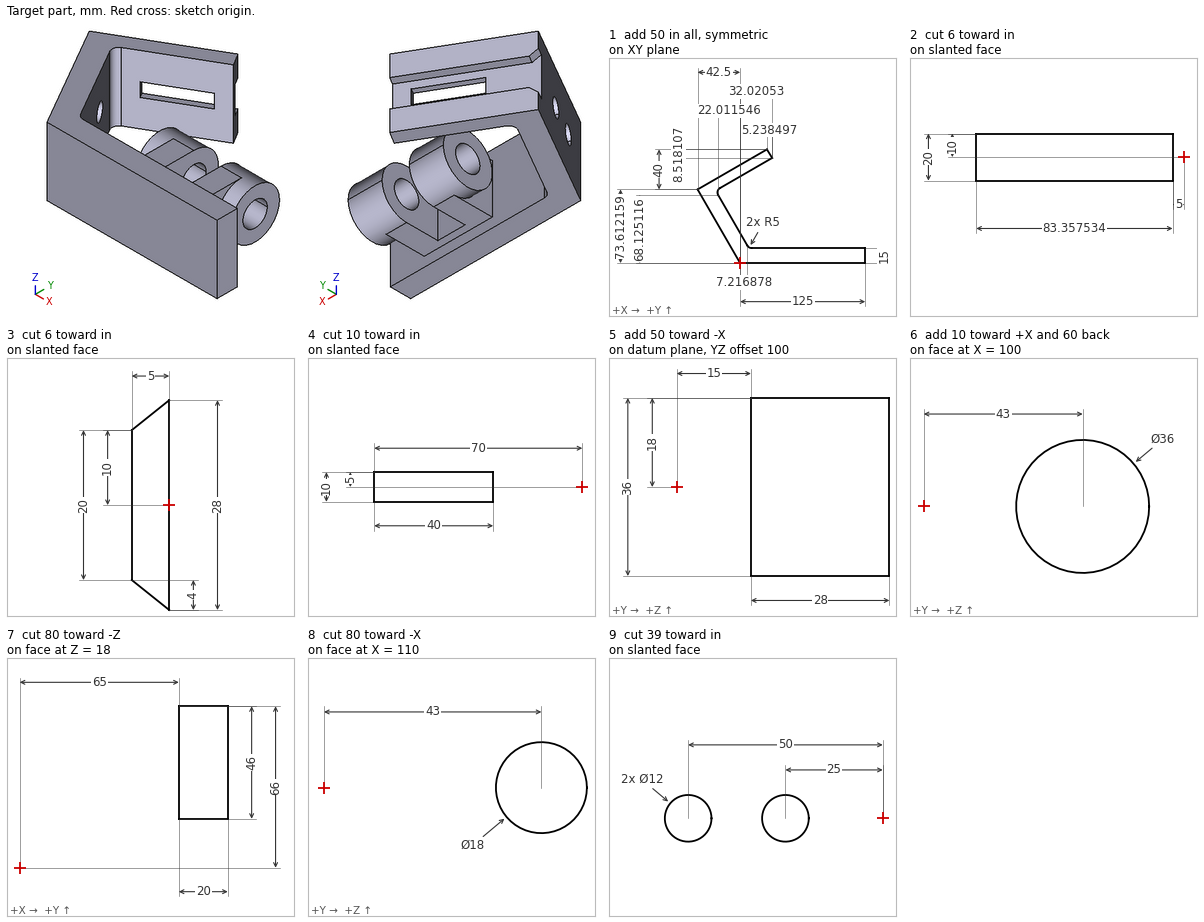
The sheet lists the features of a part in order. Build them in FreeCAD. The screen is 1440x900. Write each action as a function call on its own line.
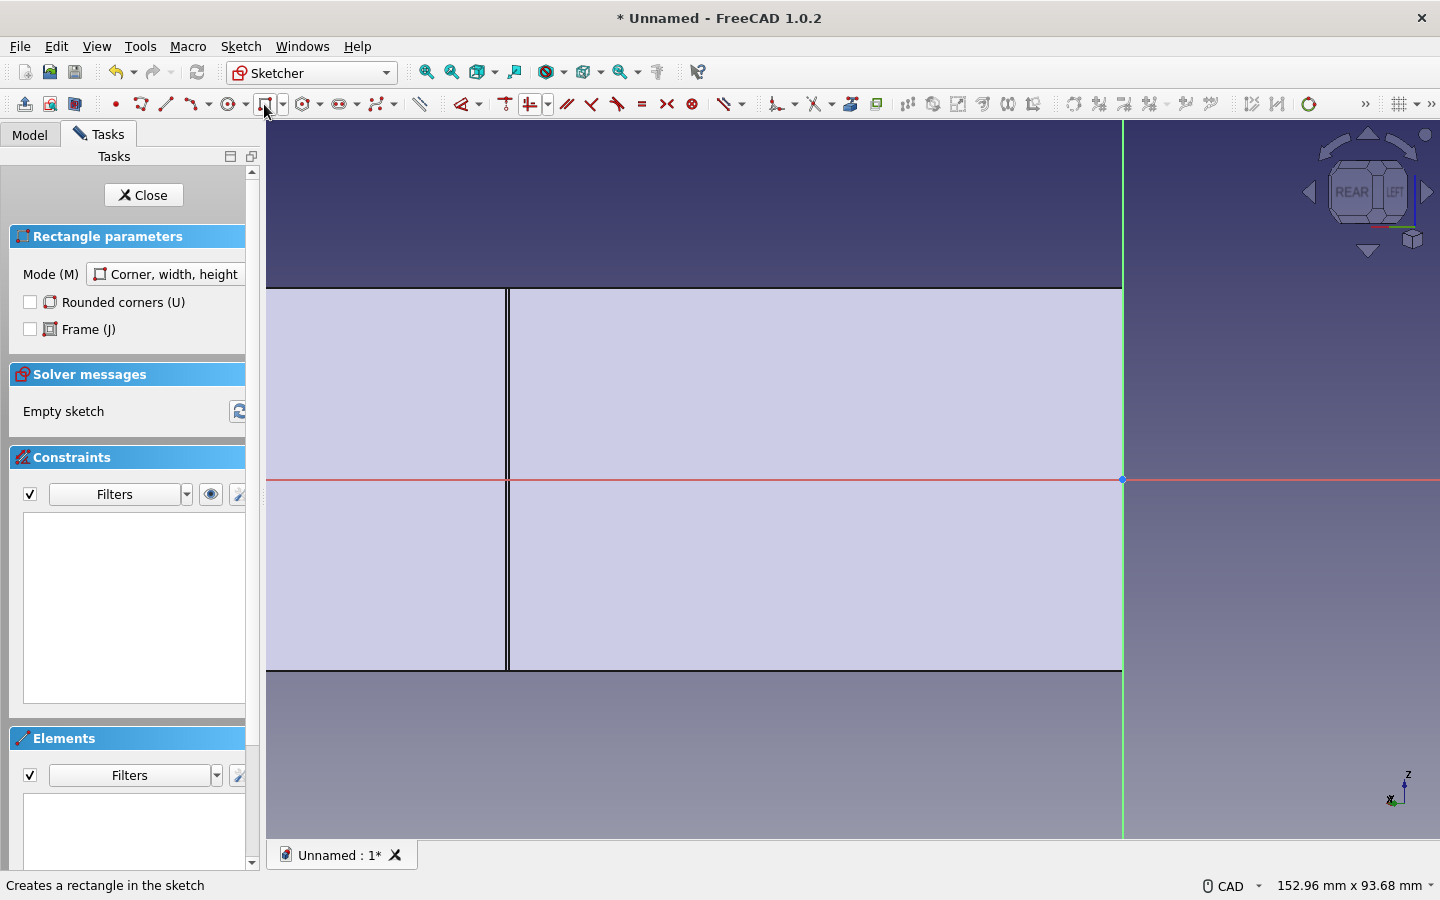
click(444, 403)
click(1084, 556)
key(Escape)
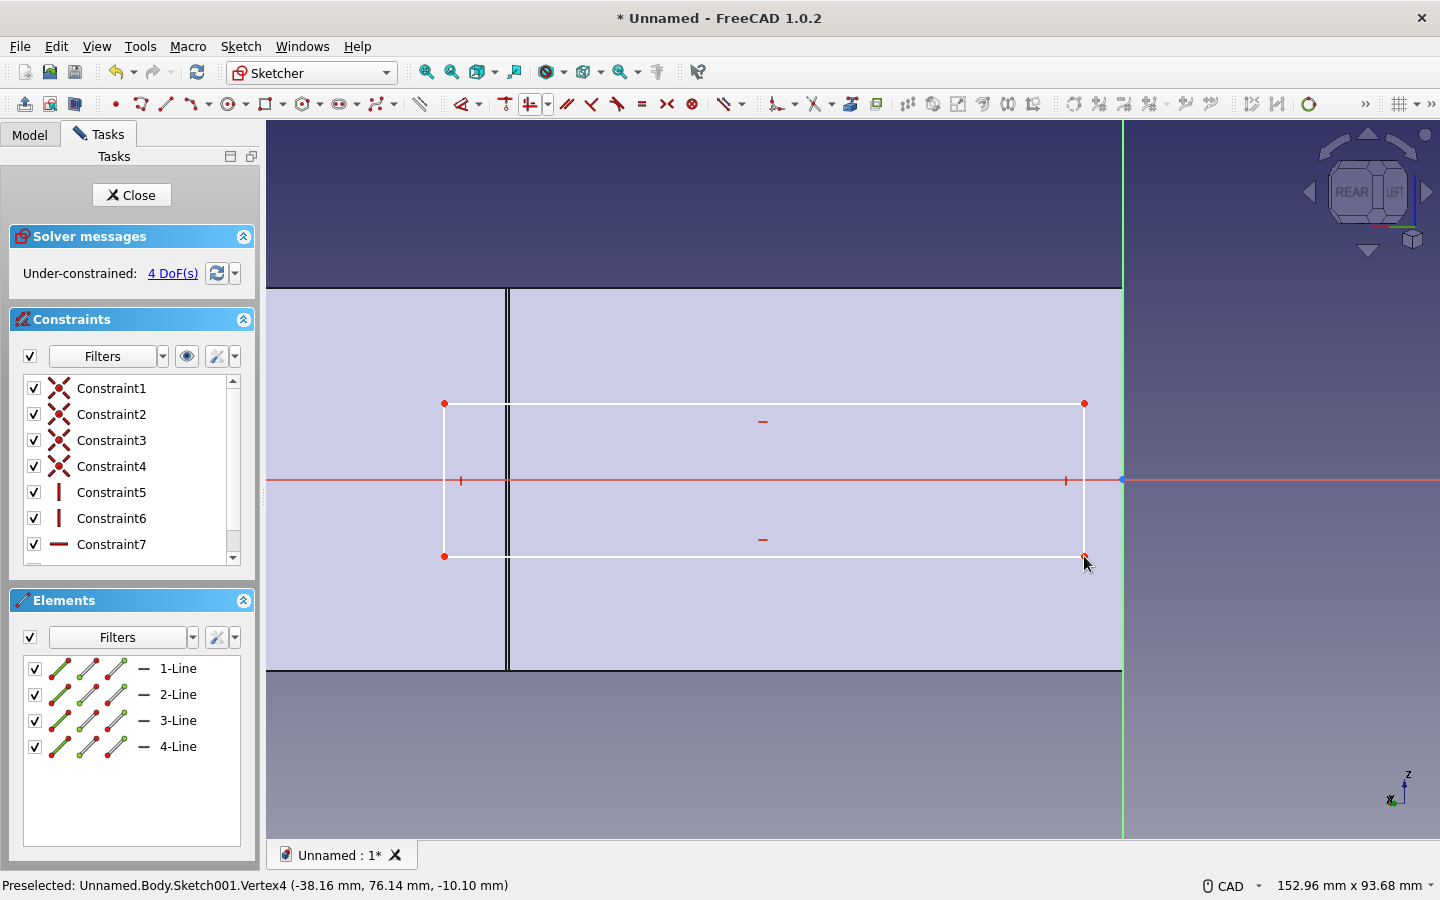
key(d)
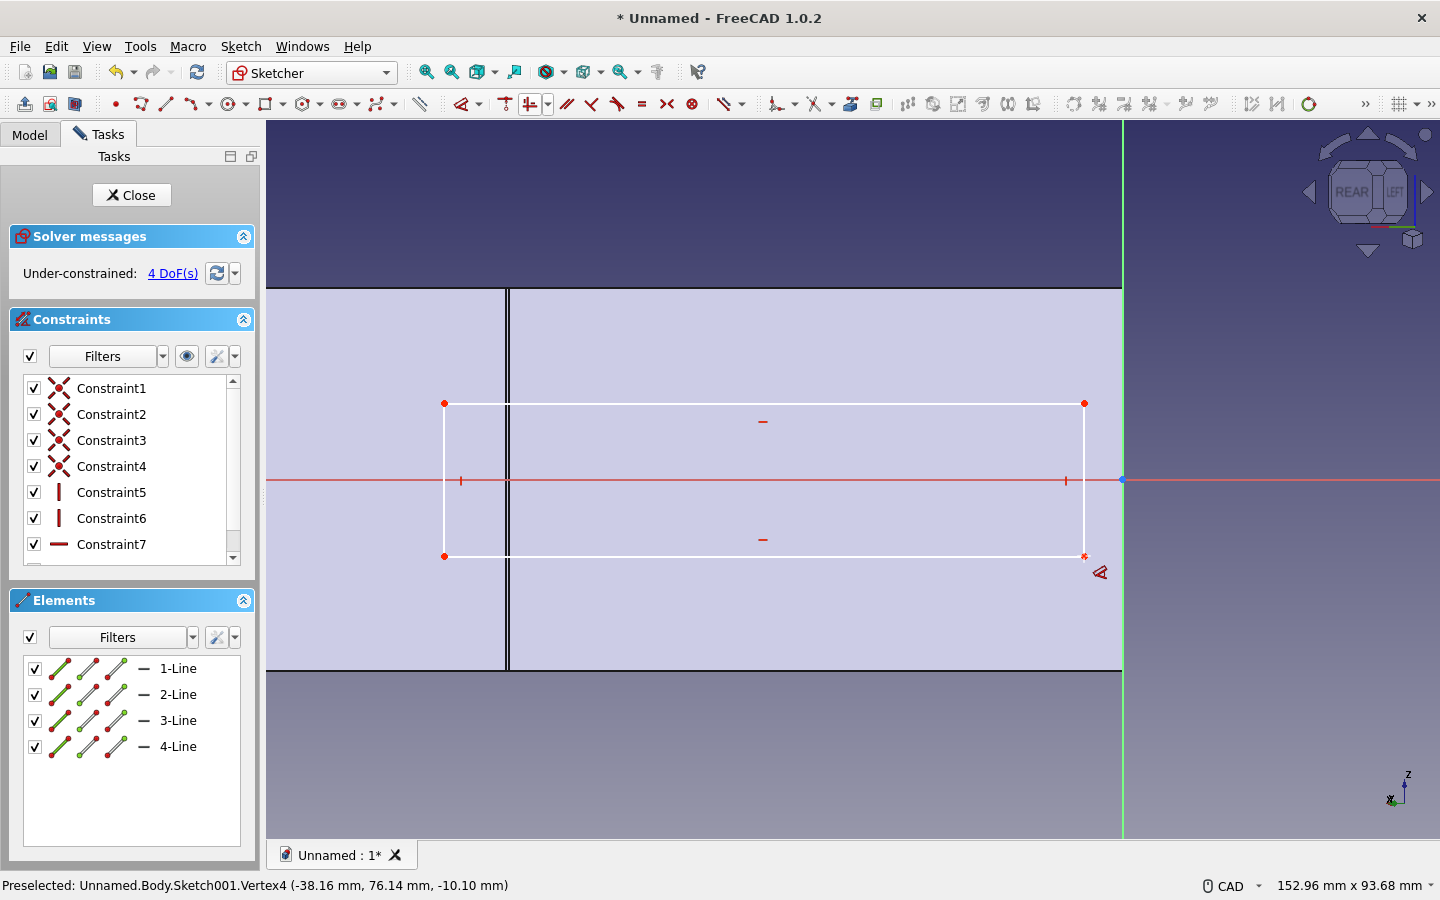
click(444, 450)
click(410, 445)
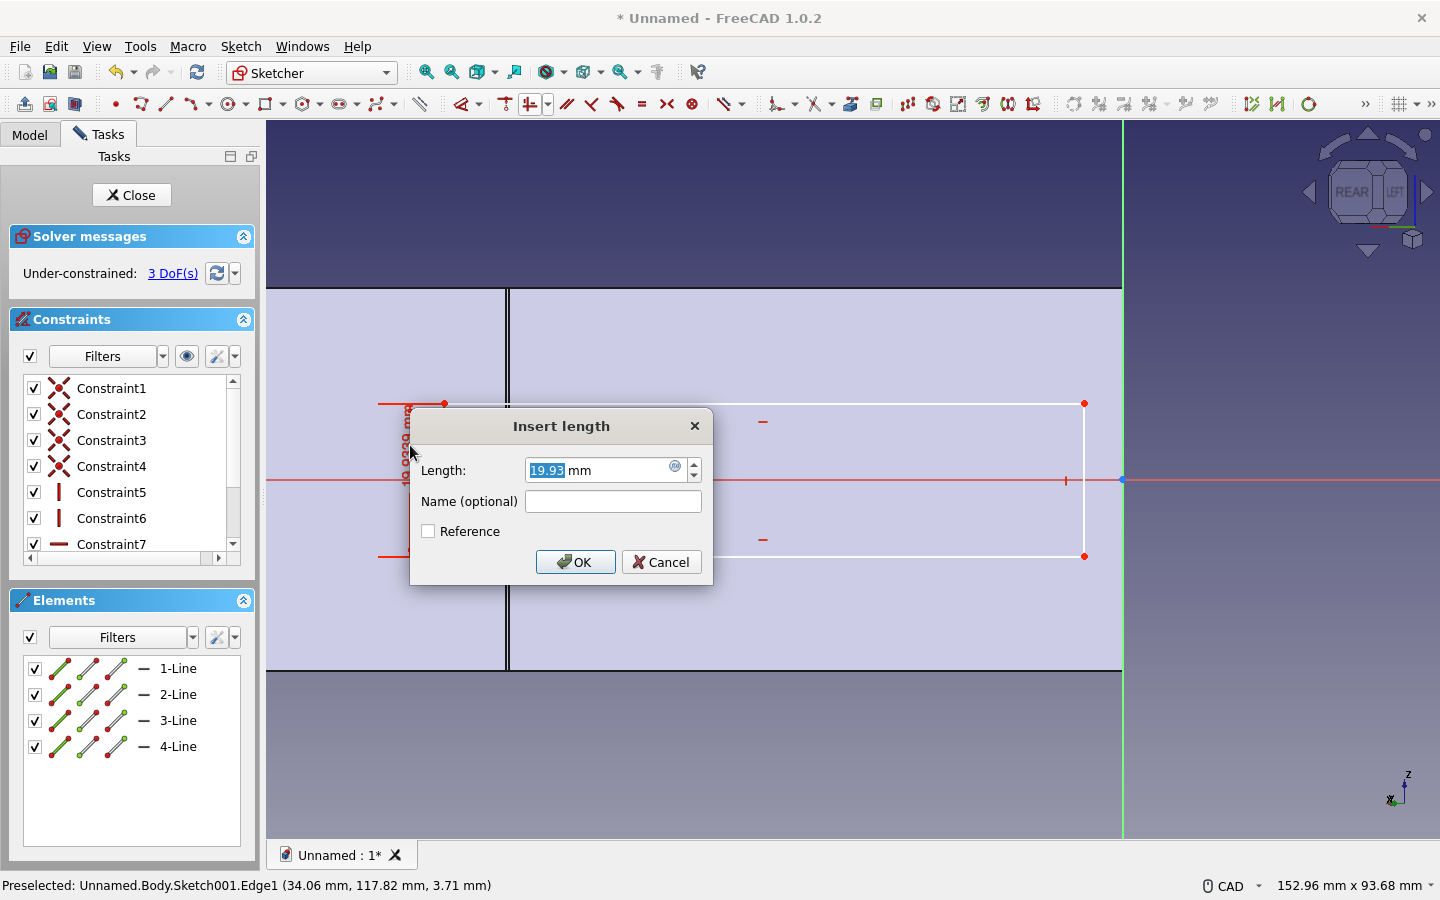
text(20)
key(Return)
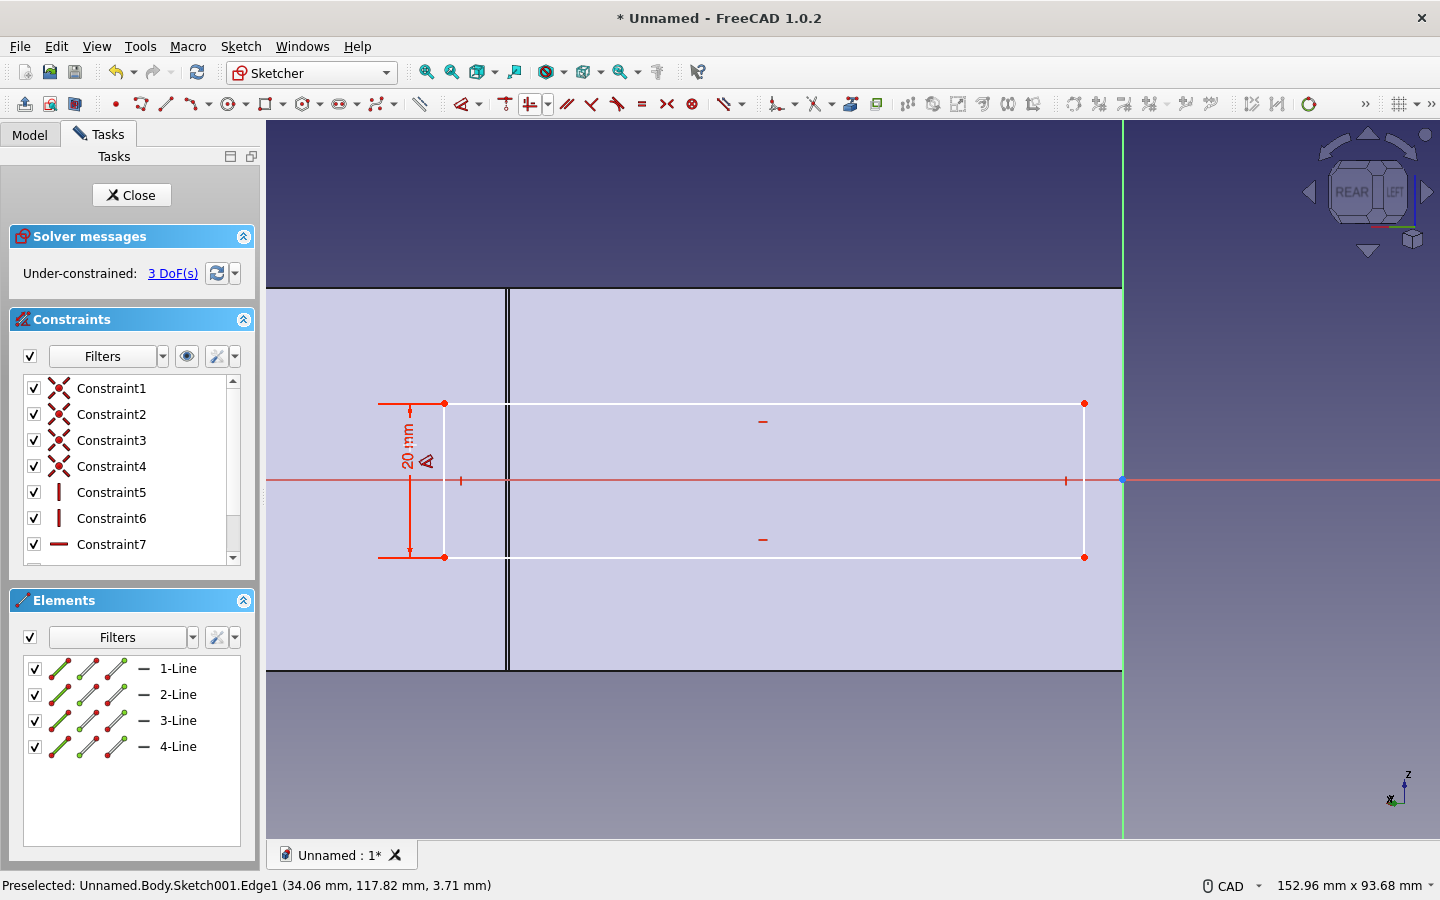
click(1084, 558)
click(1103, 592)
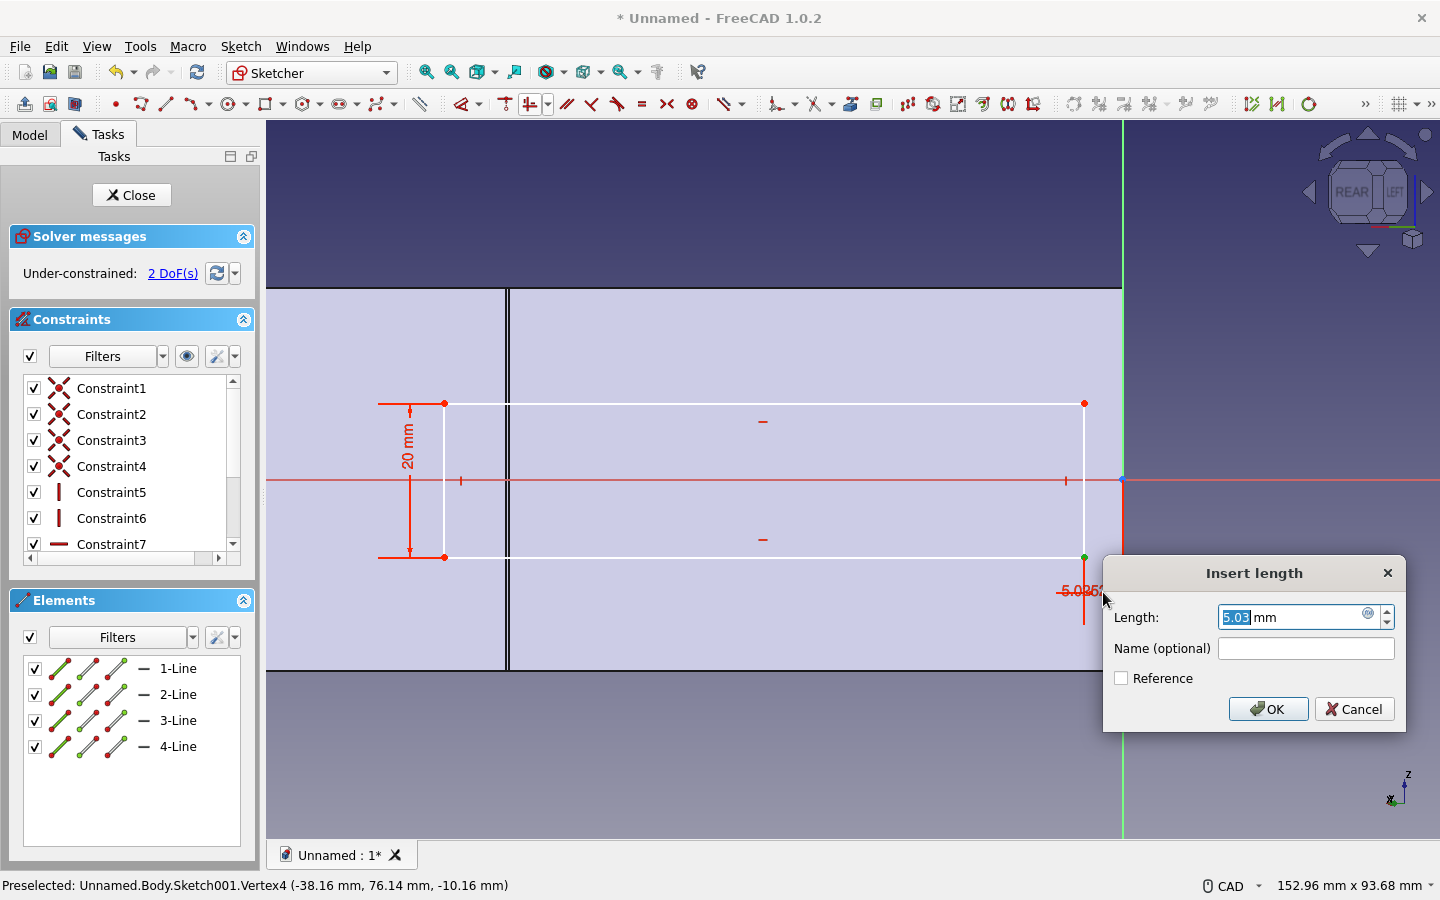
text(5)
key(Return)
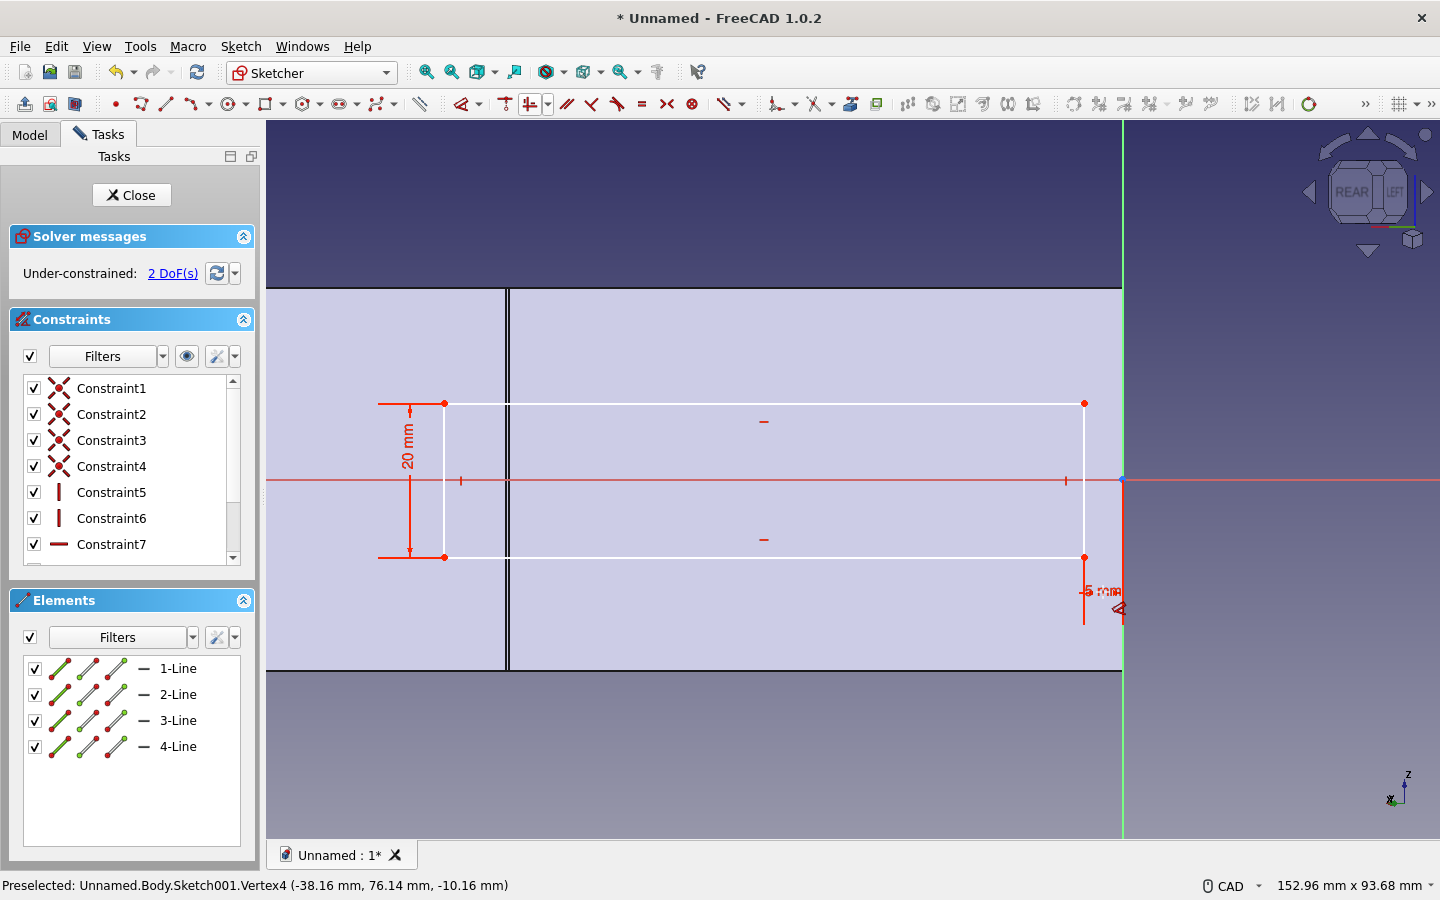
click(444, 404)
click(410, 424)